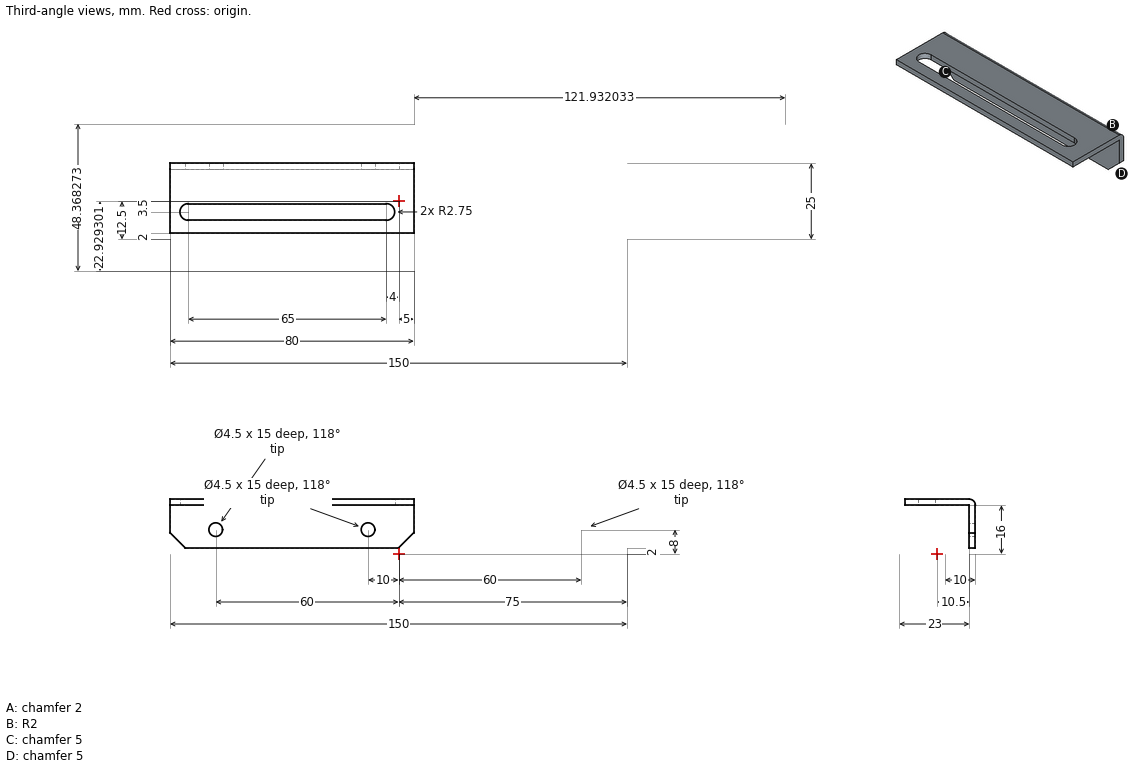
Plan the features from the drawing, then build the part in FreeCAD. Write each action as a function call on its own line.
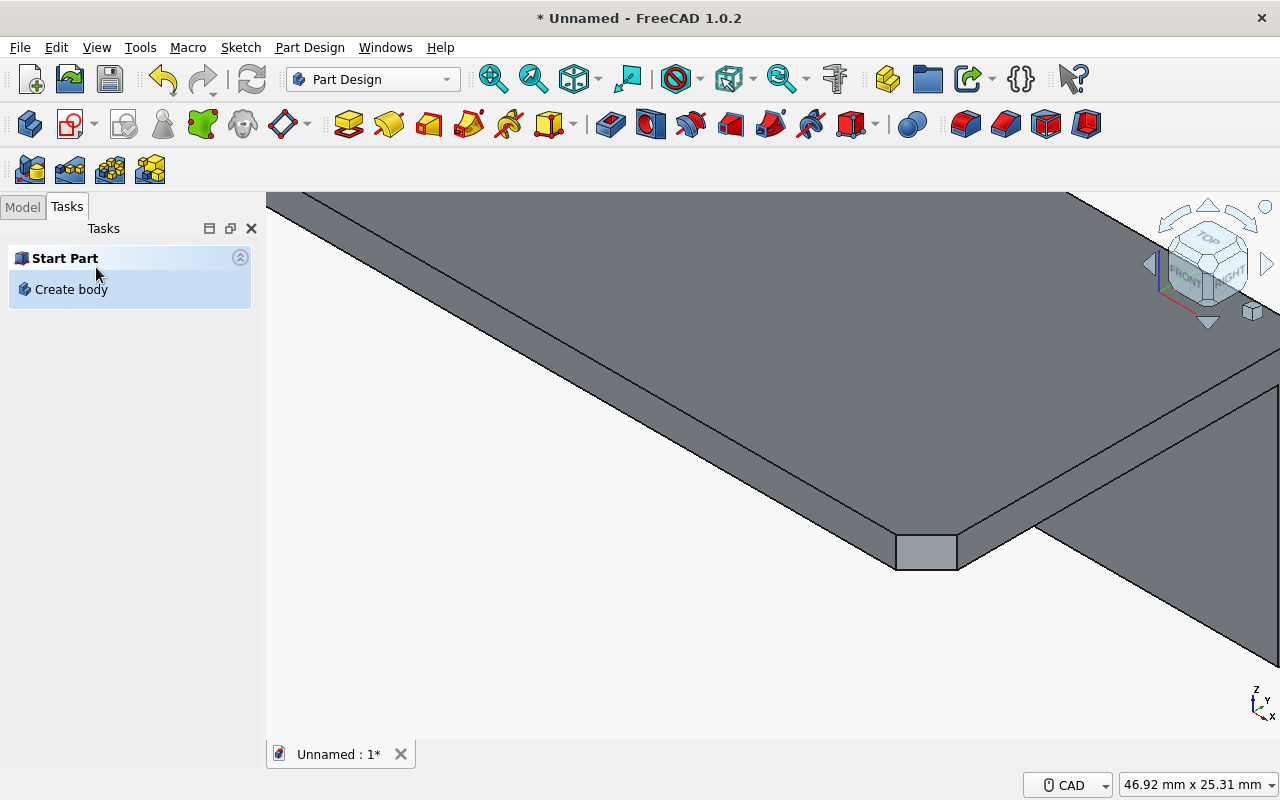
key(v)
key(f)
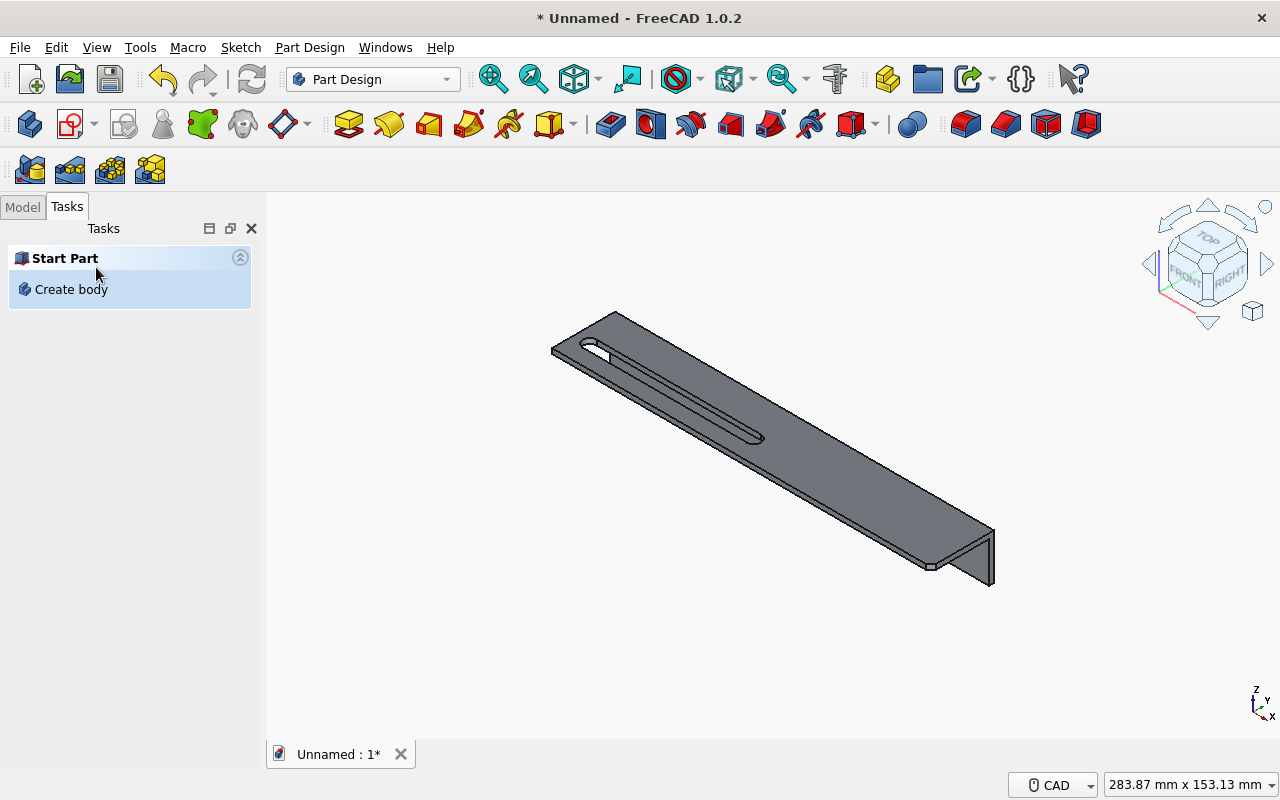
key(2)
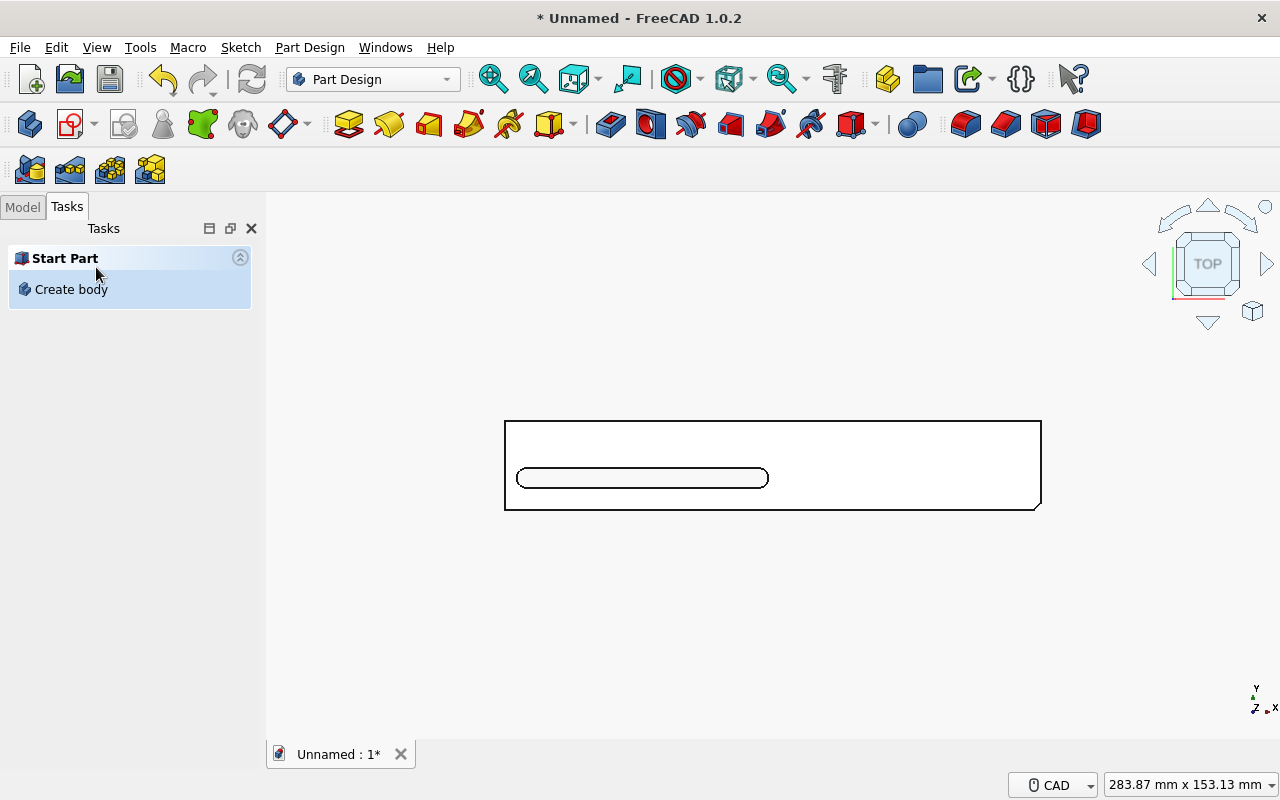
click(773, 420)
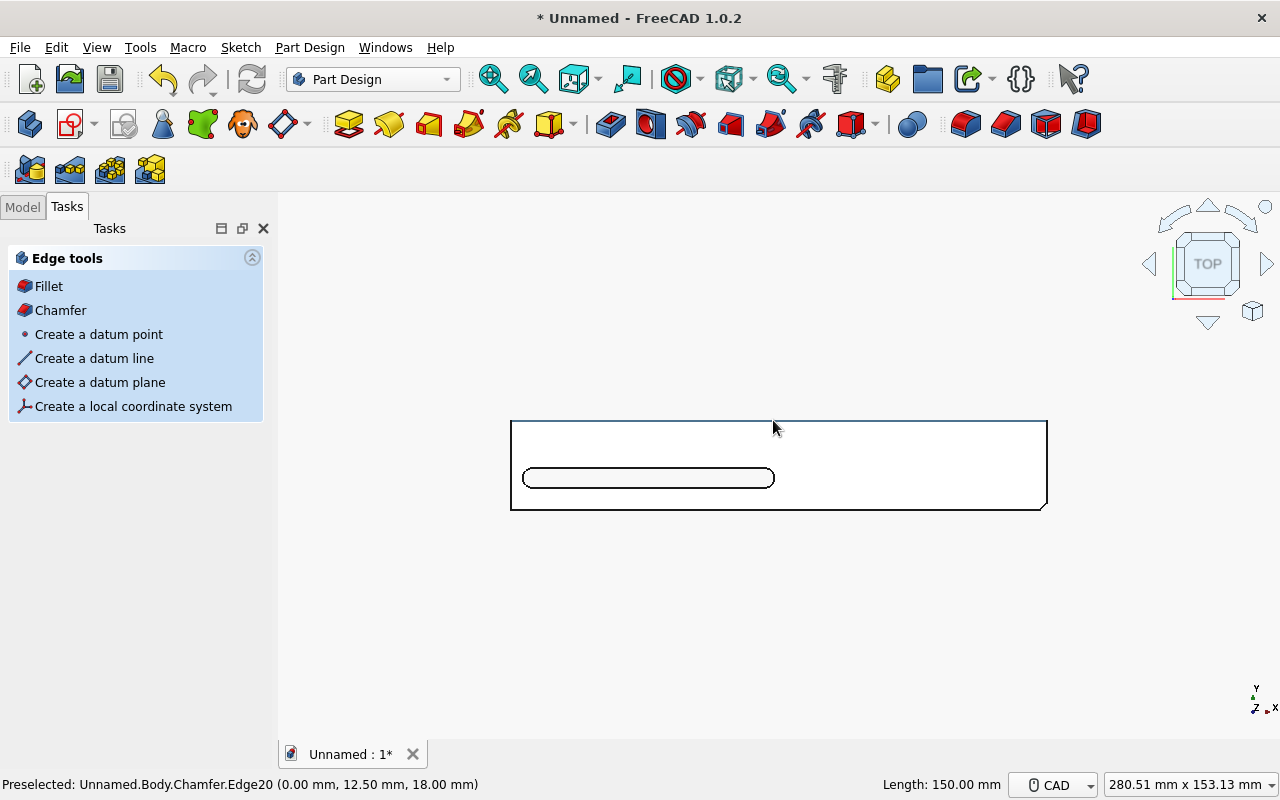
click(966, 124)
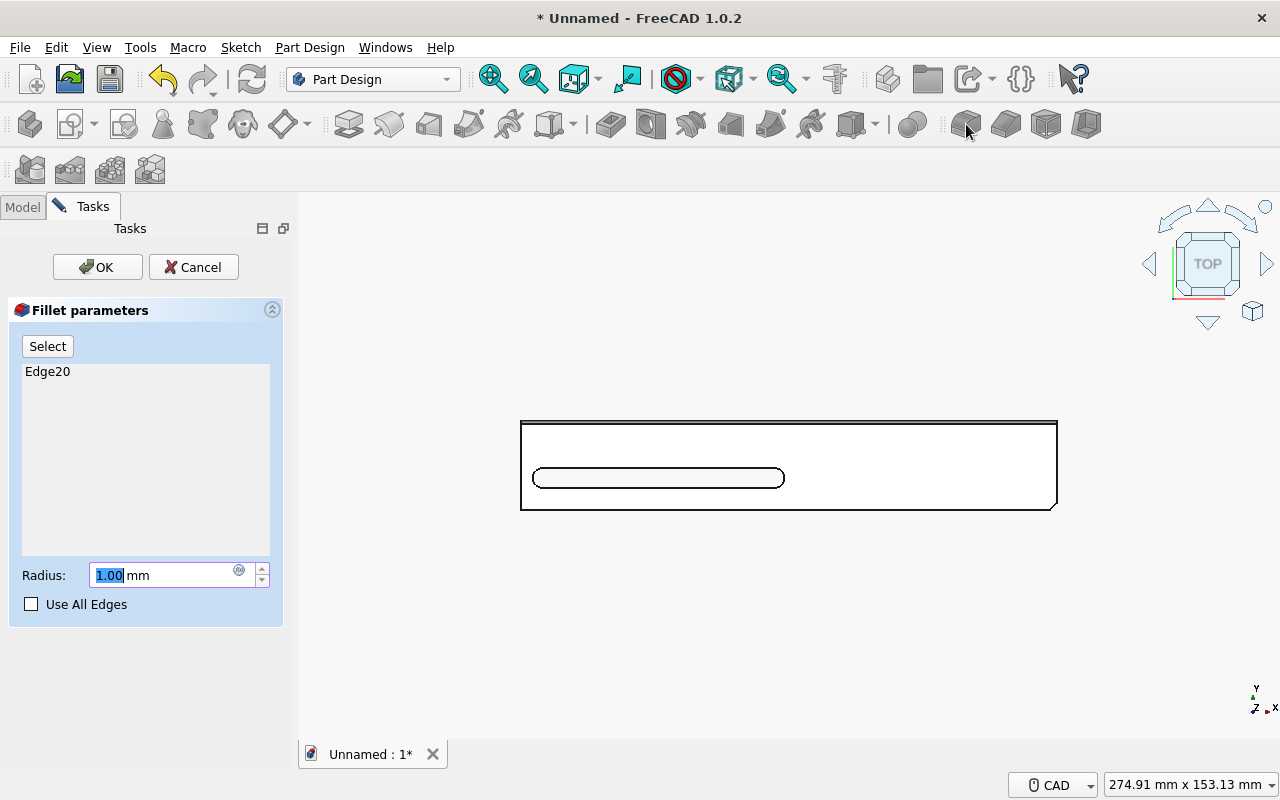
text(2)
key(Tab)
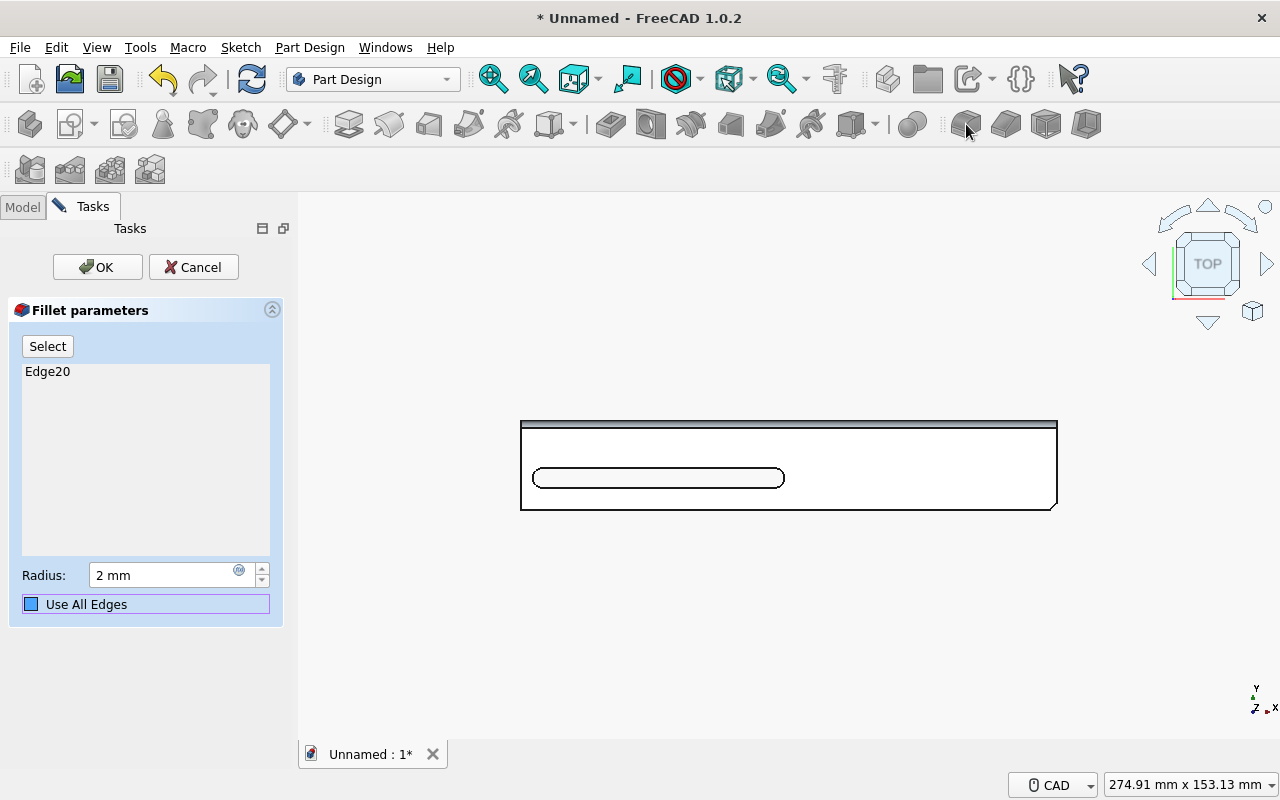
click(98, 267)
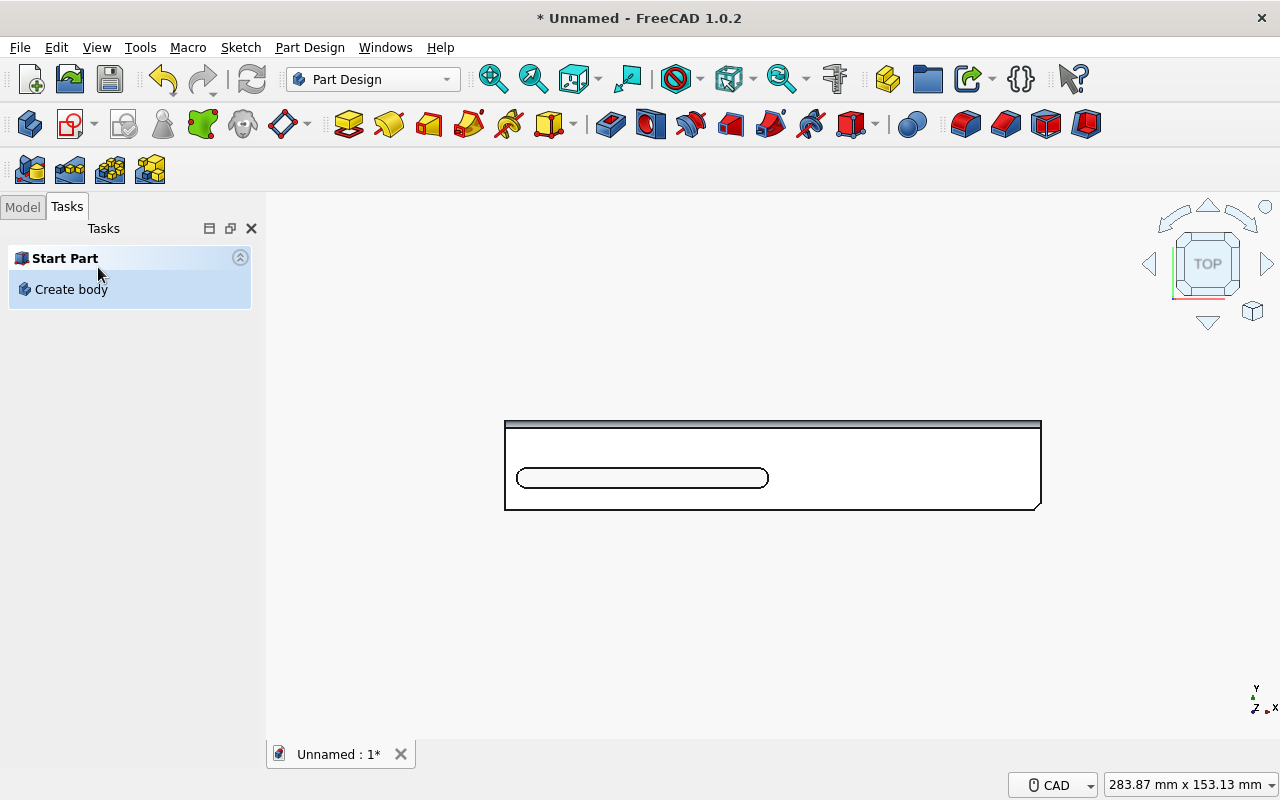
key(4)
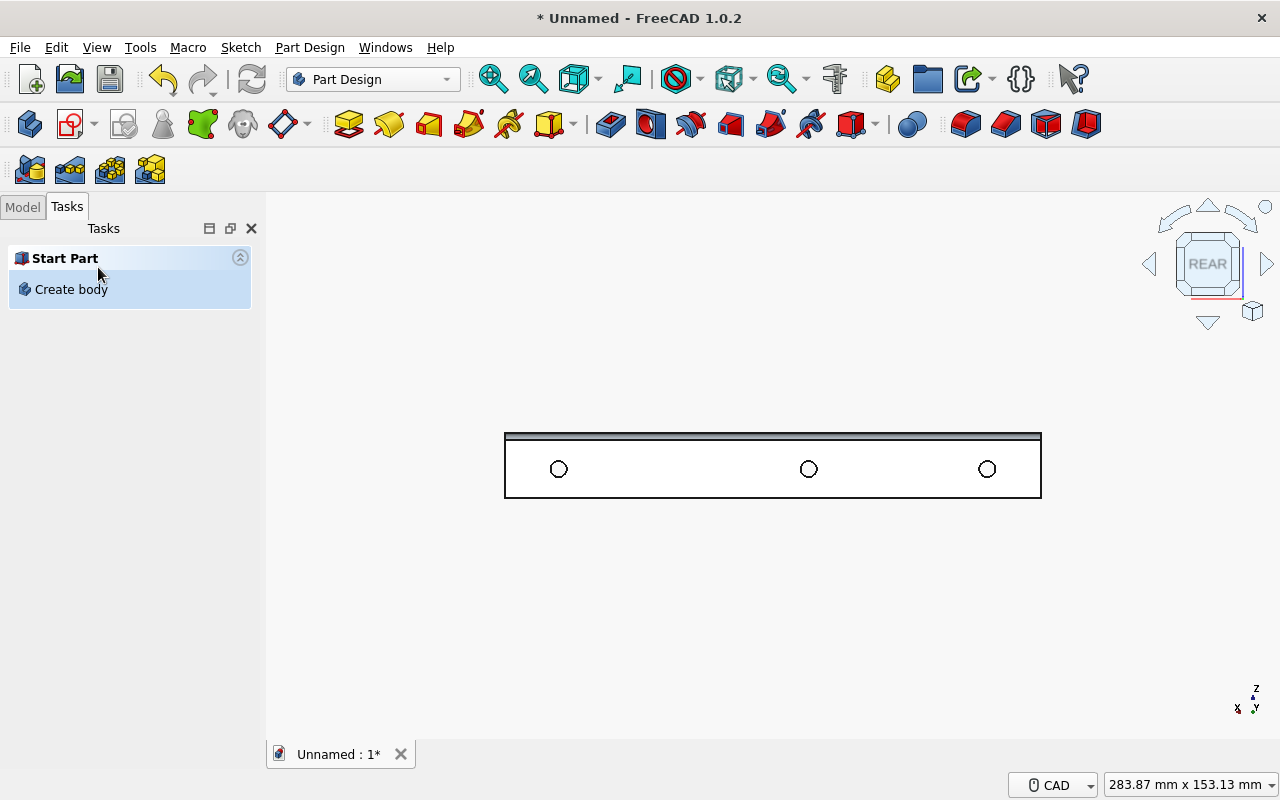
click(620, 468)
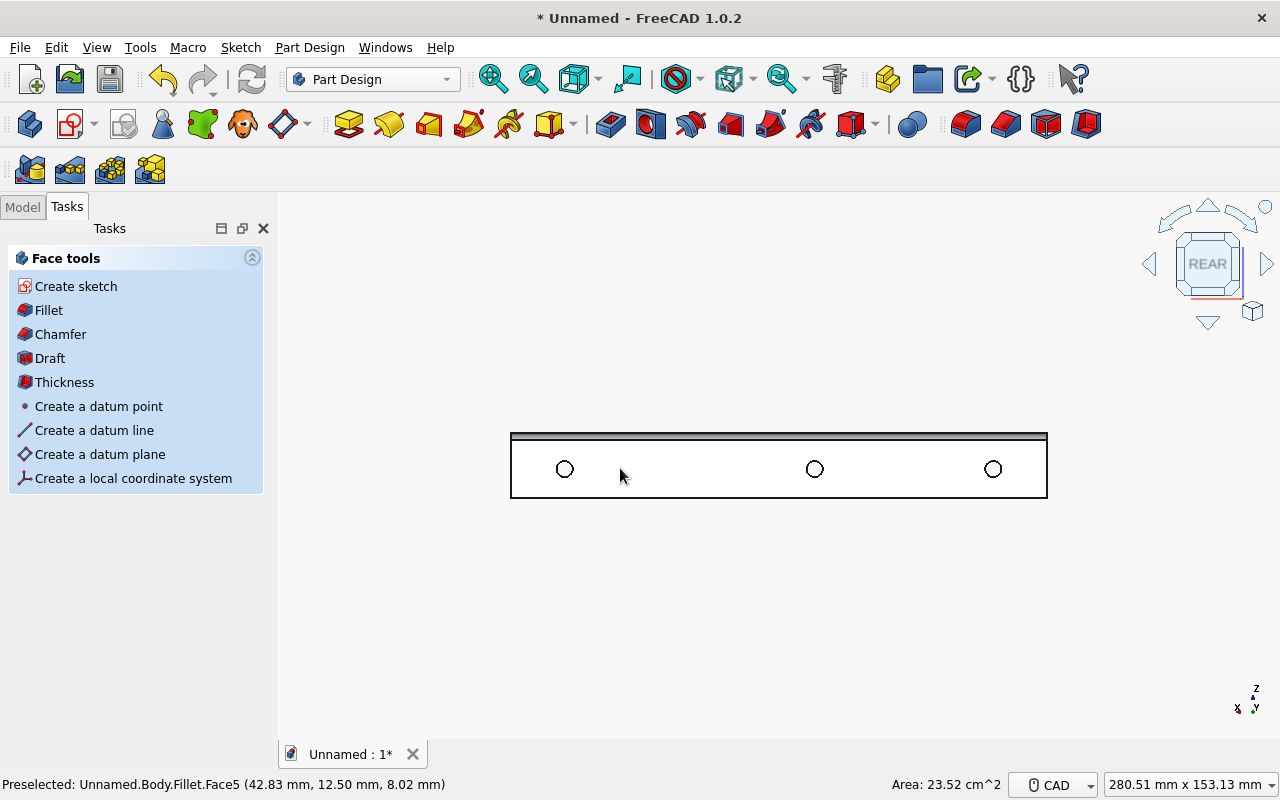
click(70, 124)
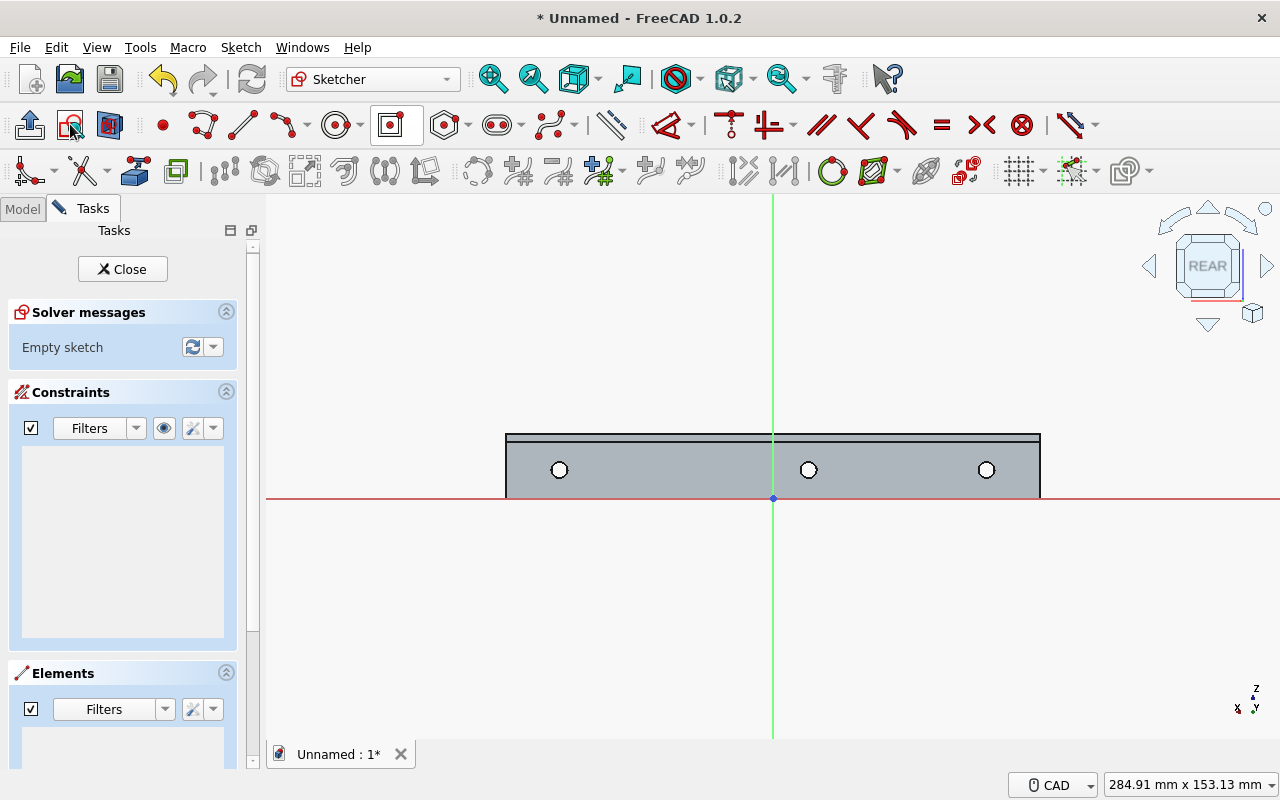
click(418, 126)